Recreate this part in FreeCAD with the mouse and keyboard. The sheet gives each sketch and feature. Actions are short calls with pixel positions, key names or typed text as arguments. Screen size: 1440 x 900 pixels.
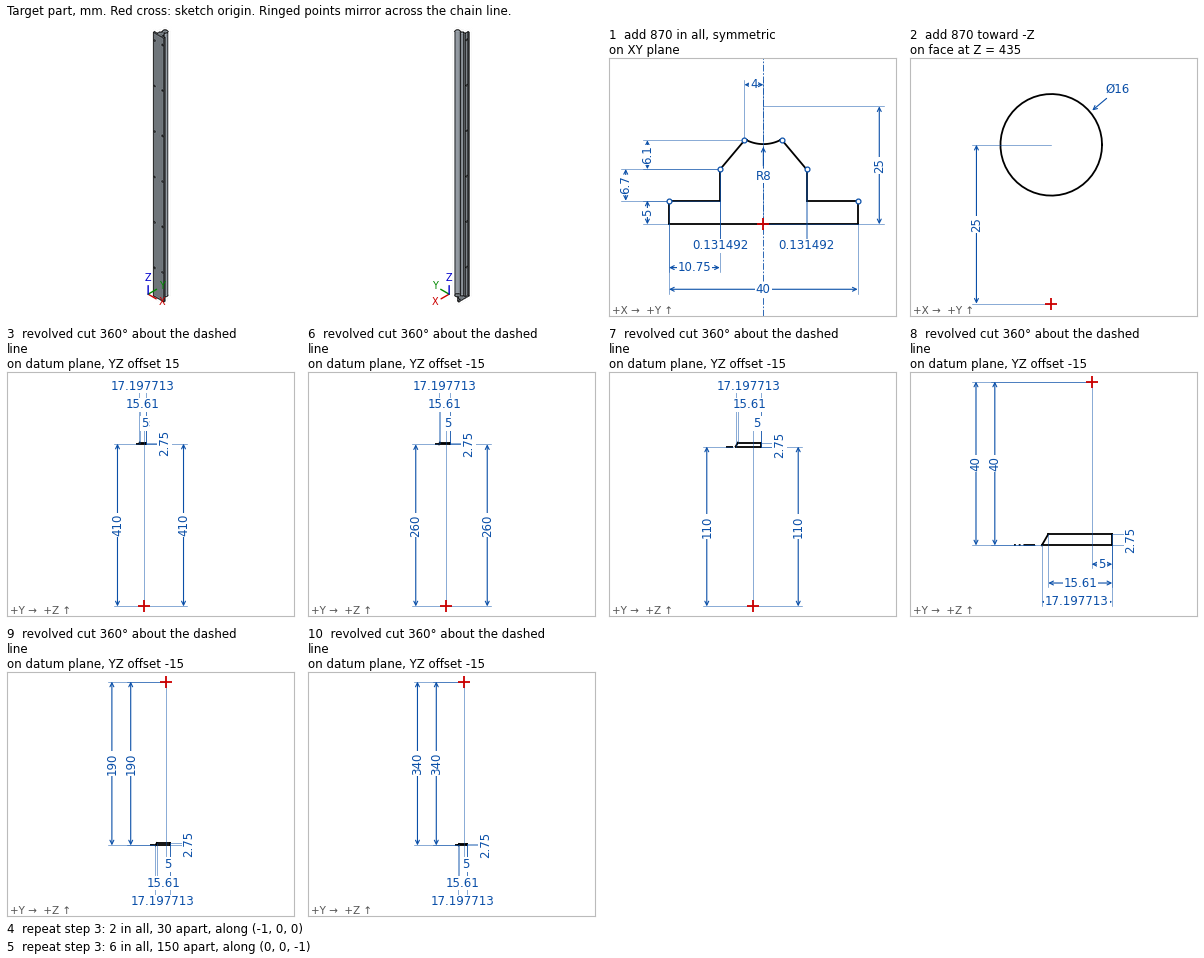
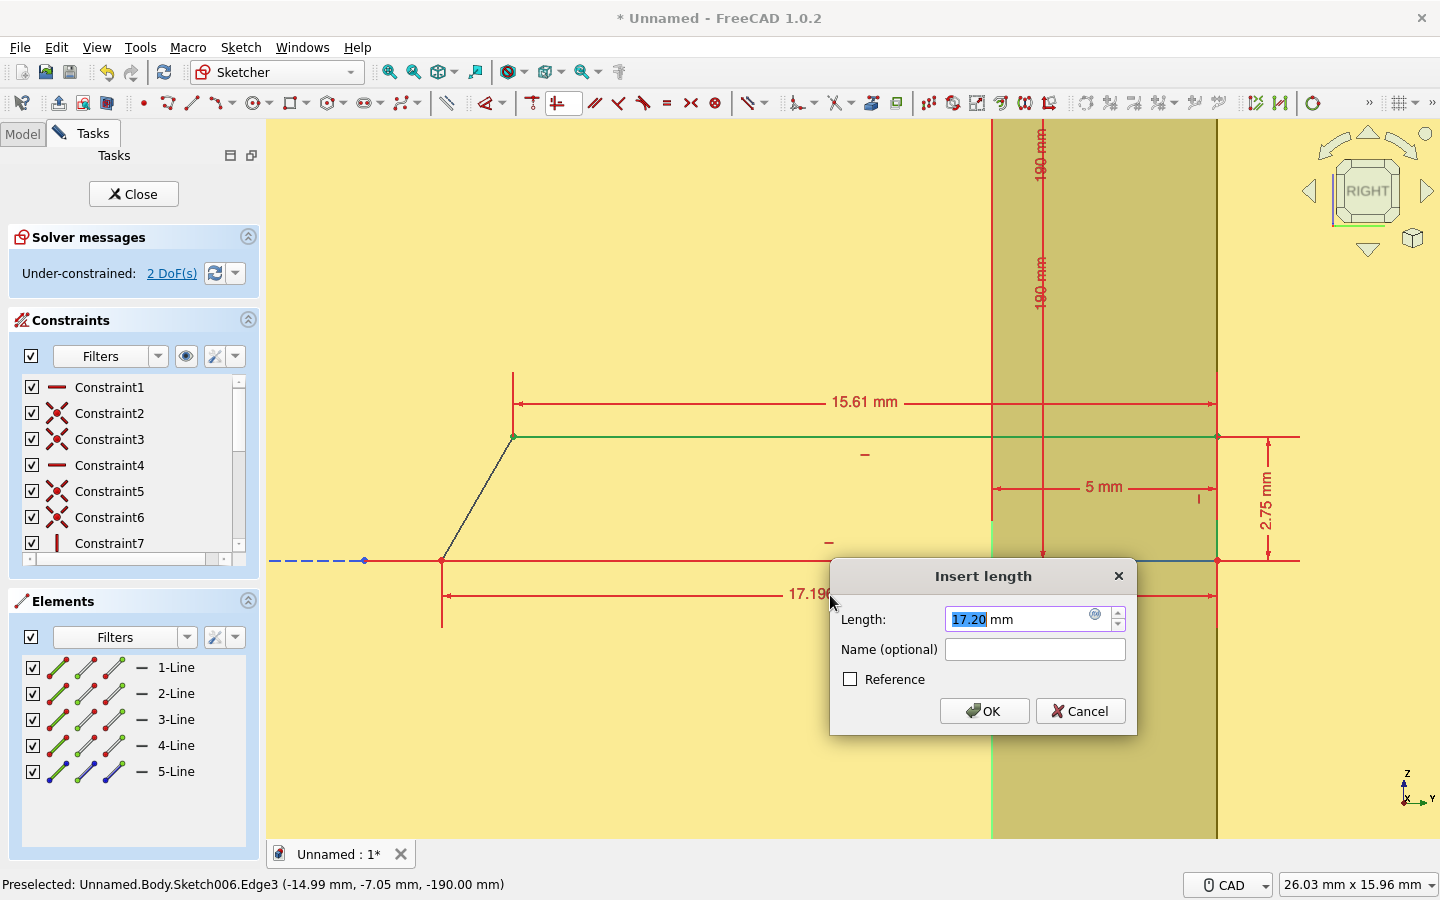
text(17.197713)
key(Return)
key(Escape)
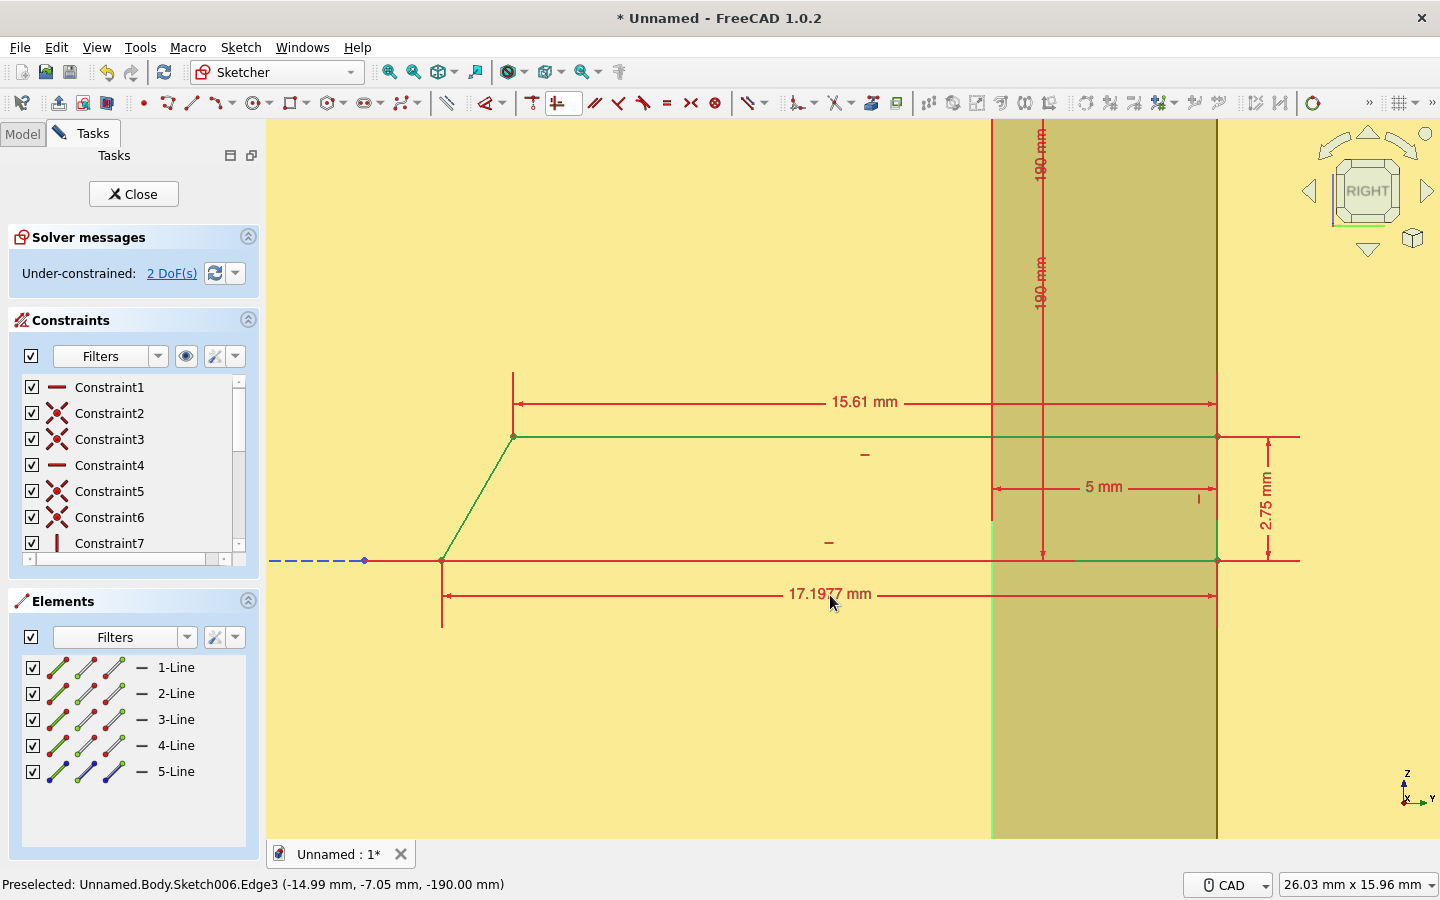
click(134, 194)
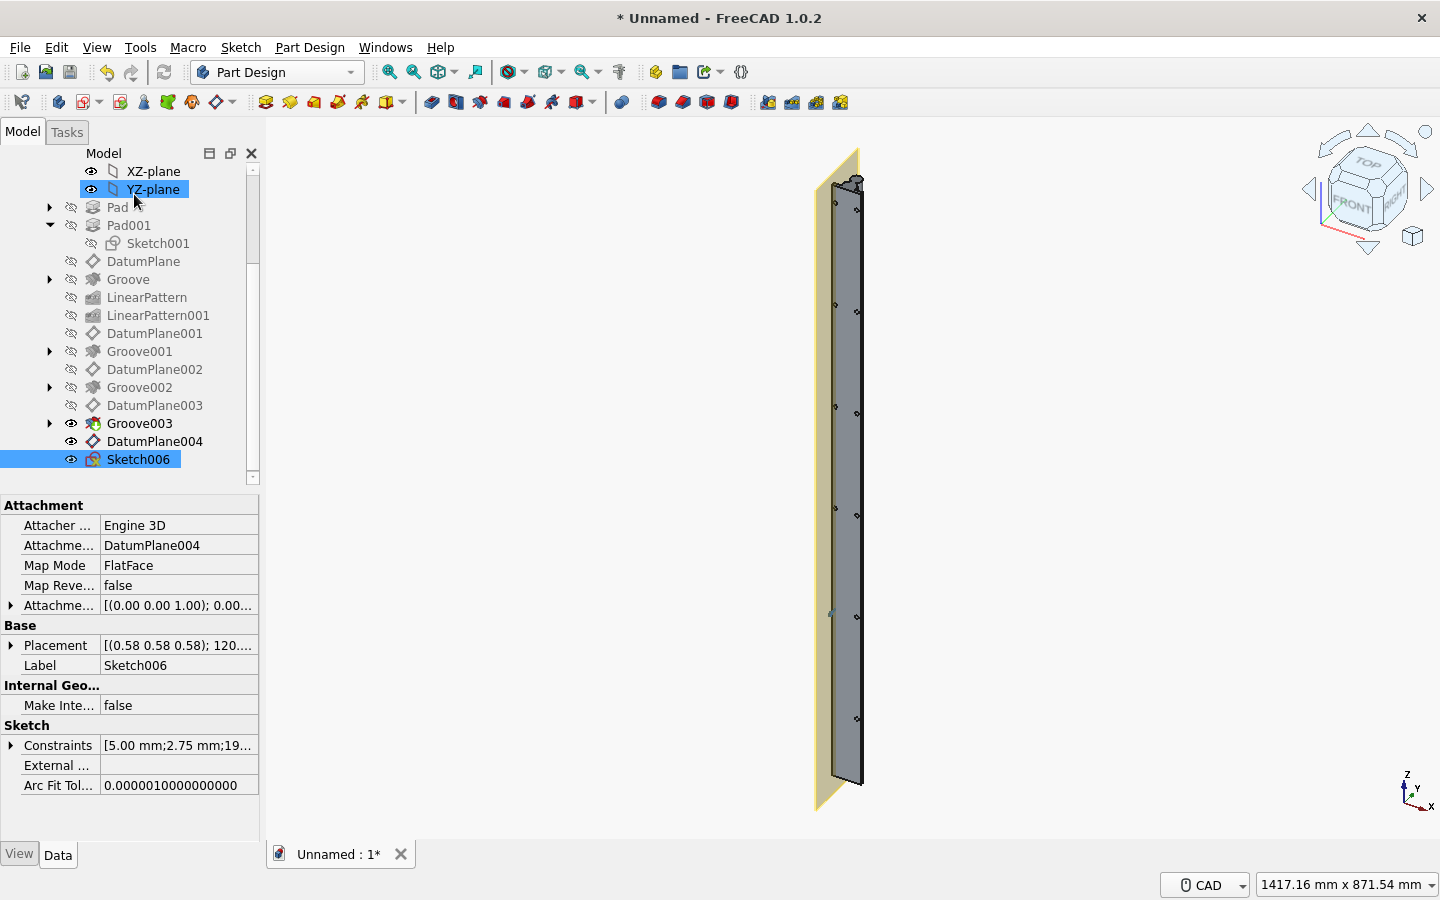
click(480, 102)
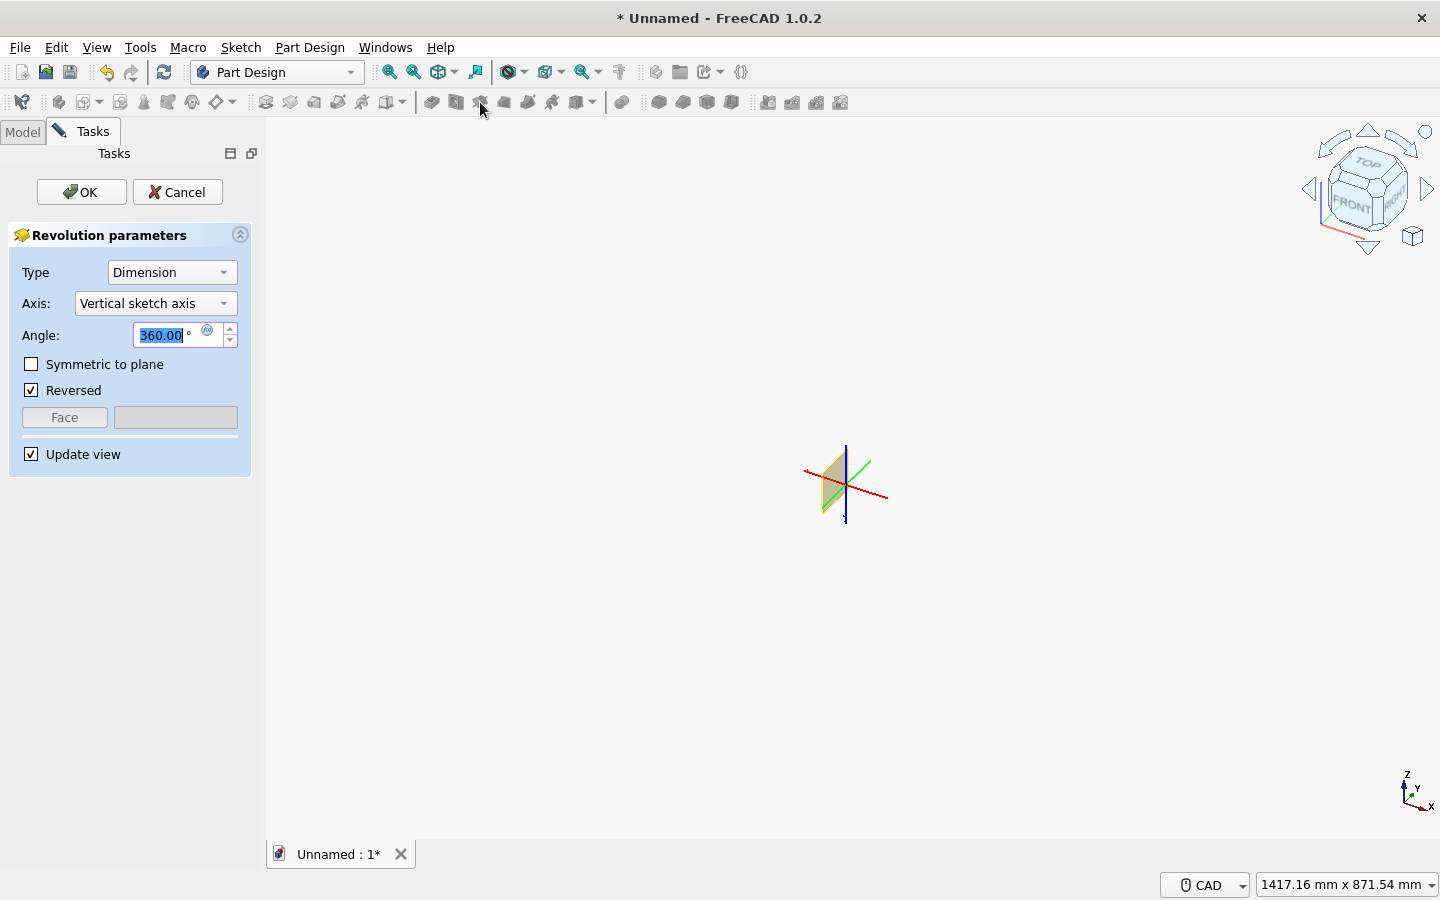
click(156, 304)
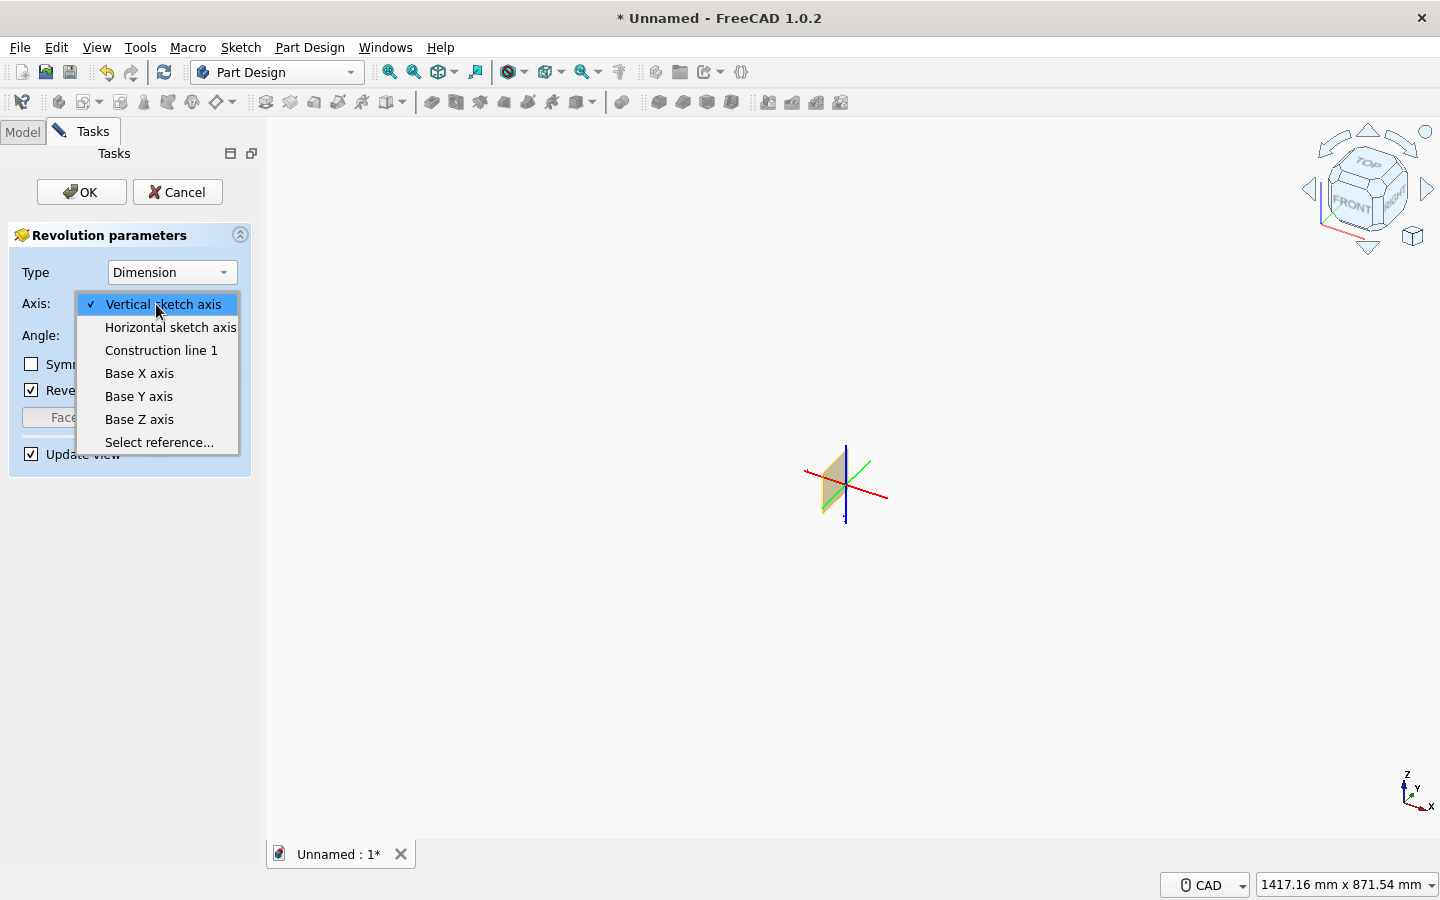
click(156, 350)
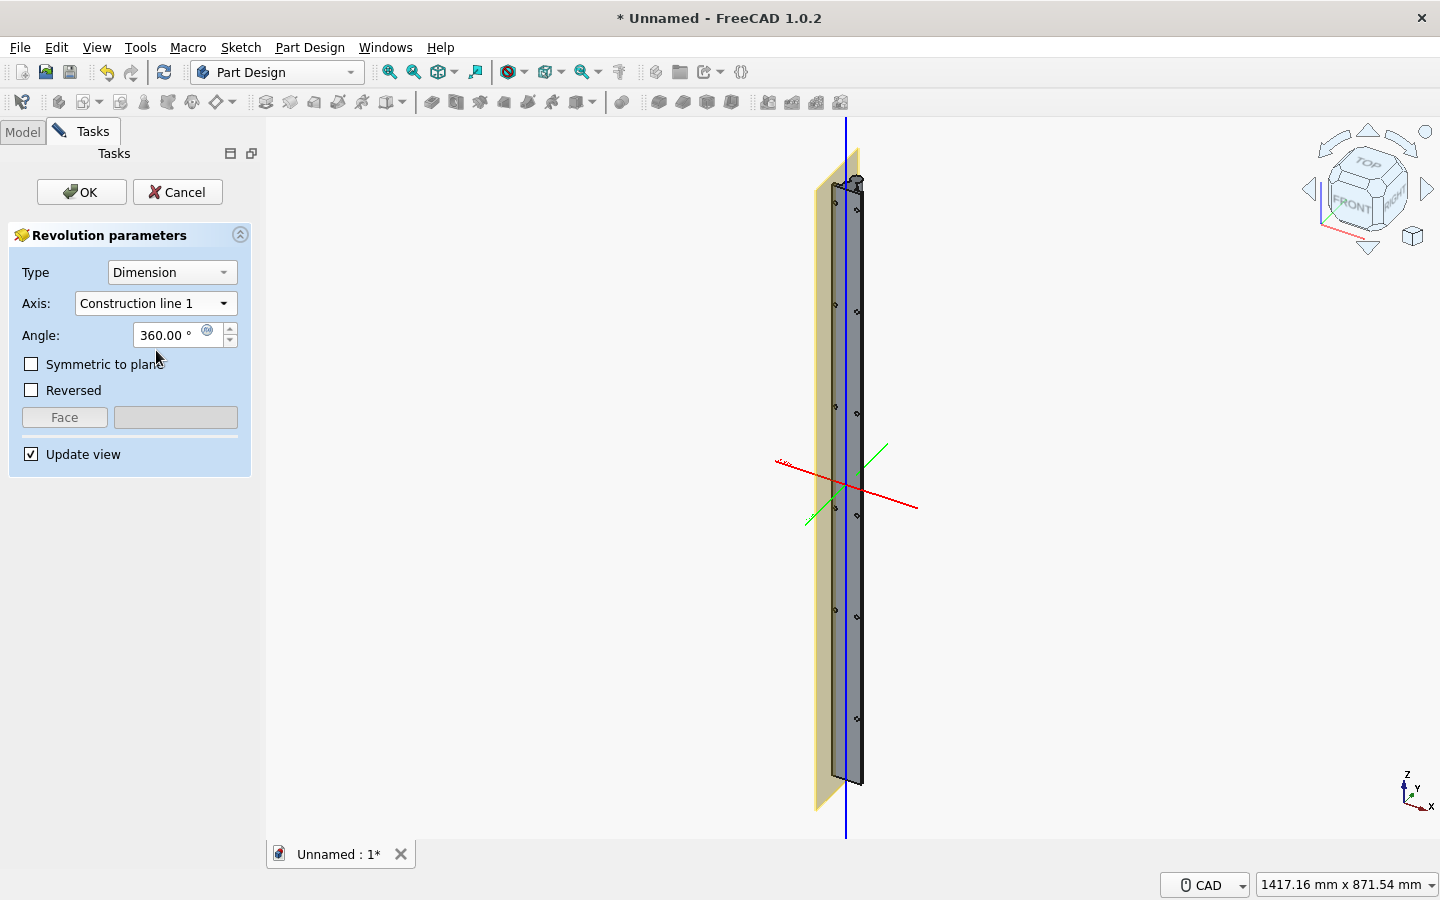
click(82, 192)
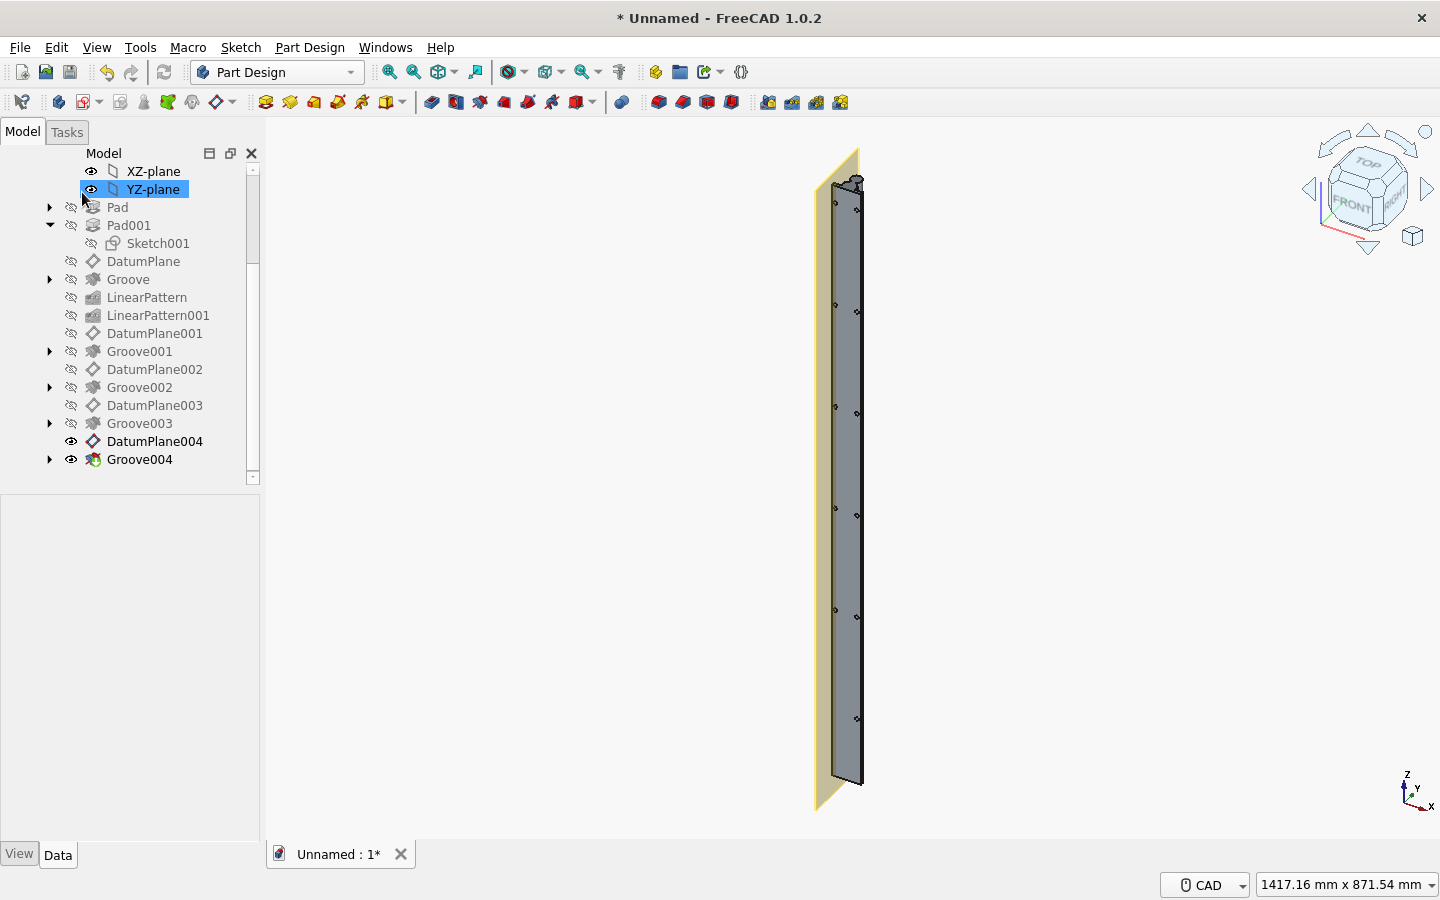
click(116, 441)
key(space)